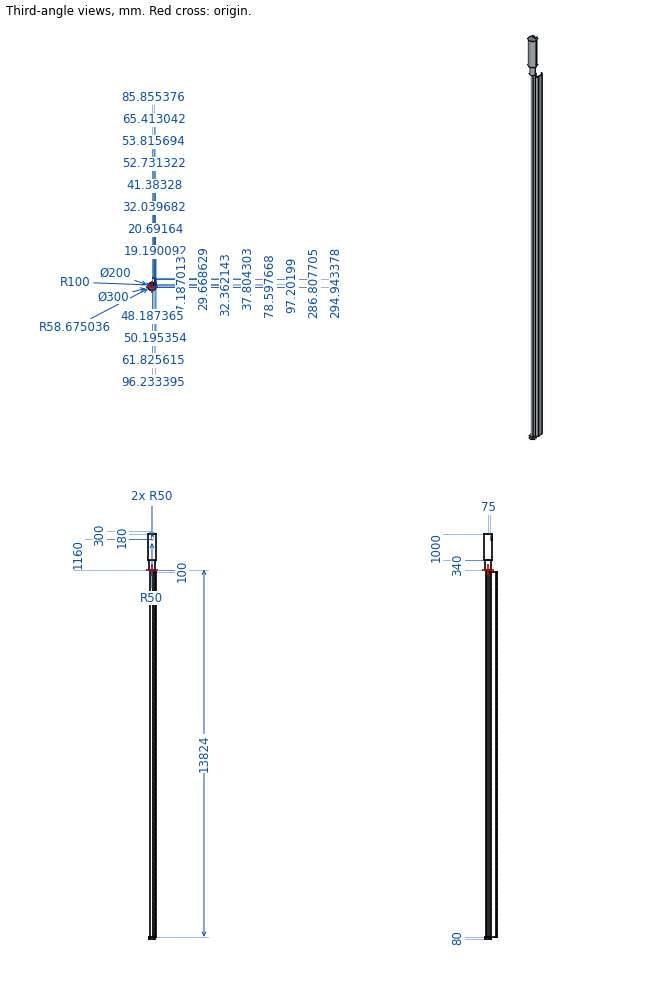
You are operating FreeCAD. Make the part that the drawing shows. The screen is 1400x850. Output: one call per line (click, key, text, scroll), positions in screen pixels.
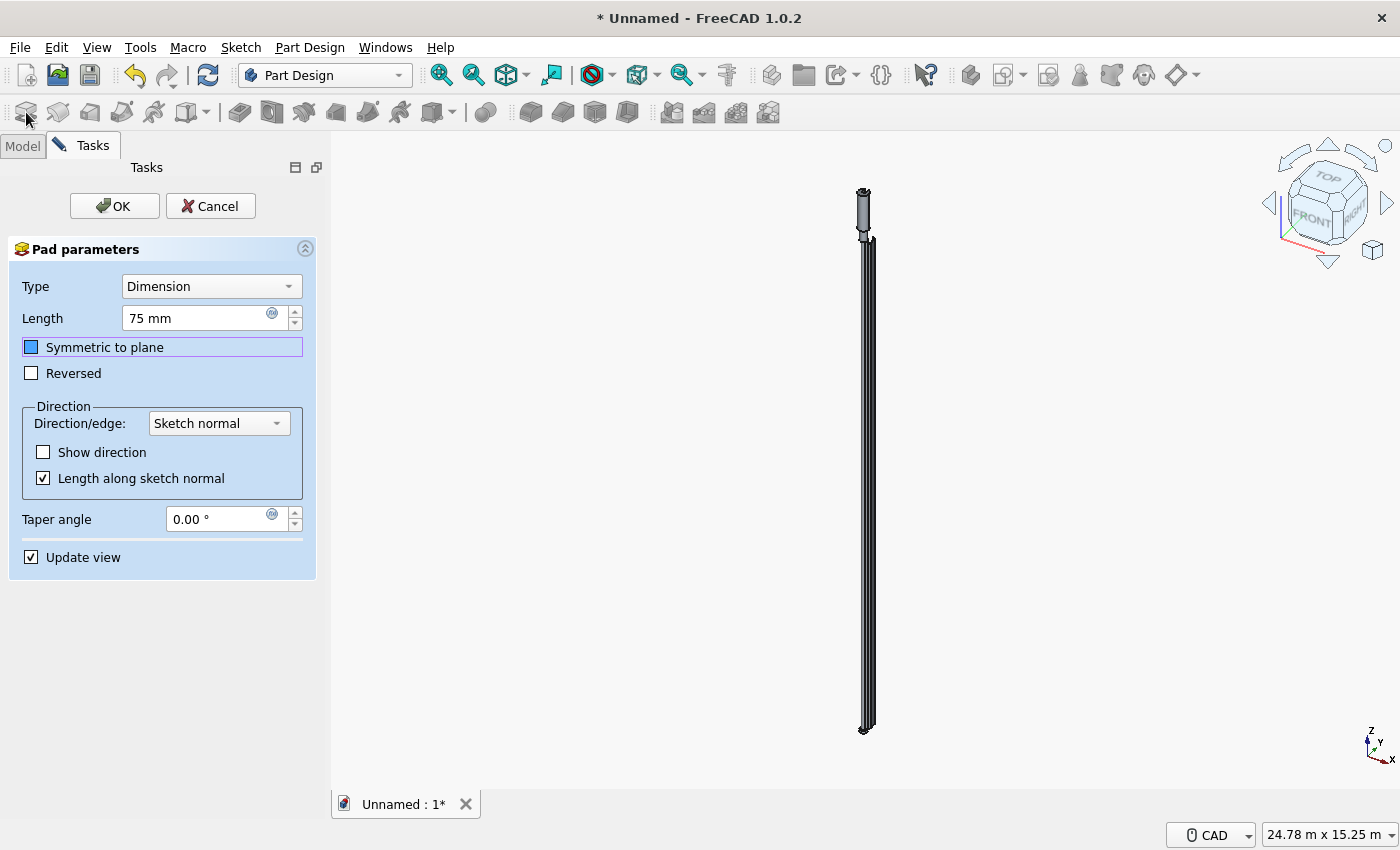
click(30, 373)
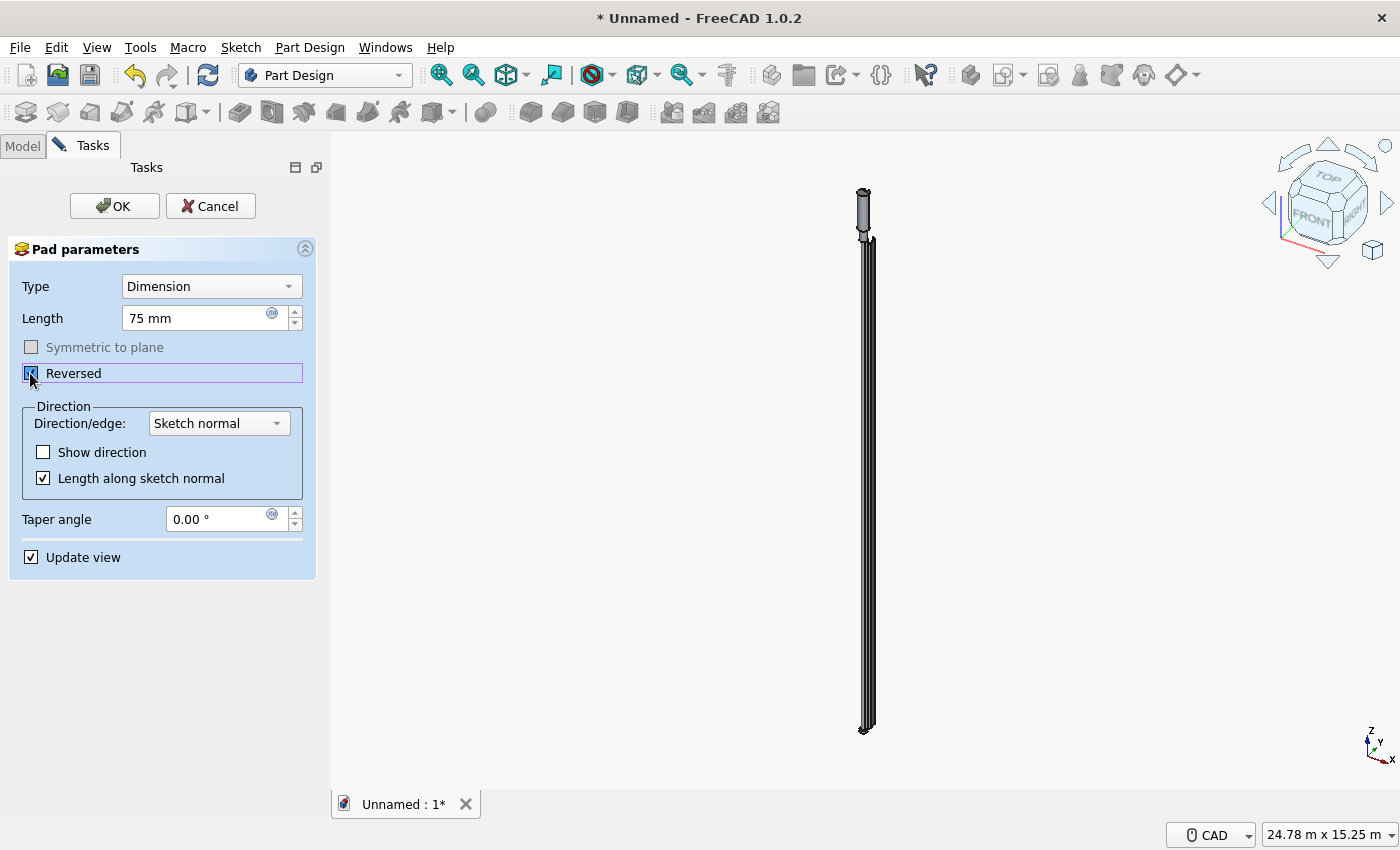
click(115, 206)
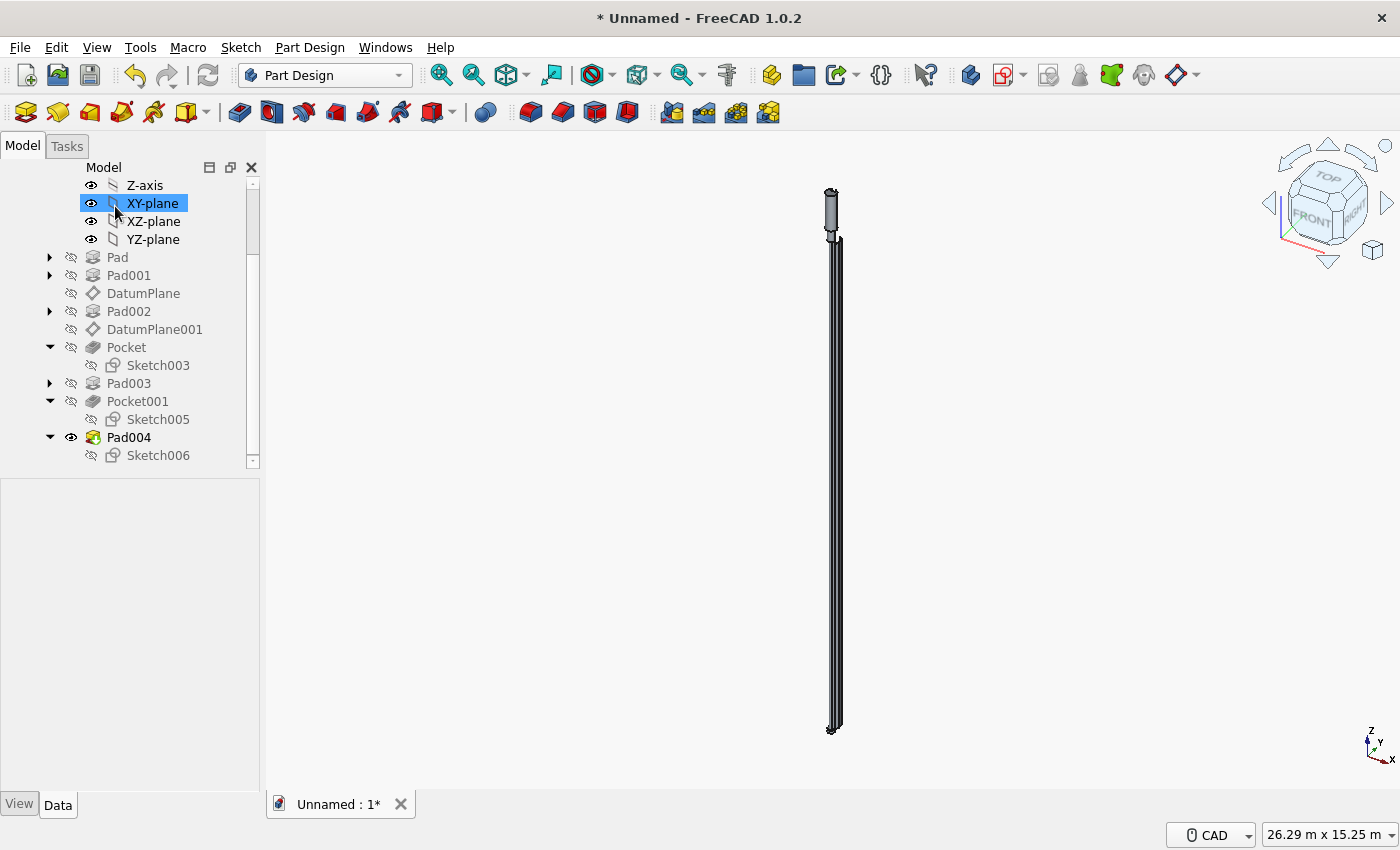
key(0)